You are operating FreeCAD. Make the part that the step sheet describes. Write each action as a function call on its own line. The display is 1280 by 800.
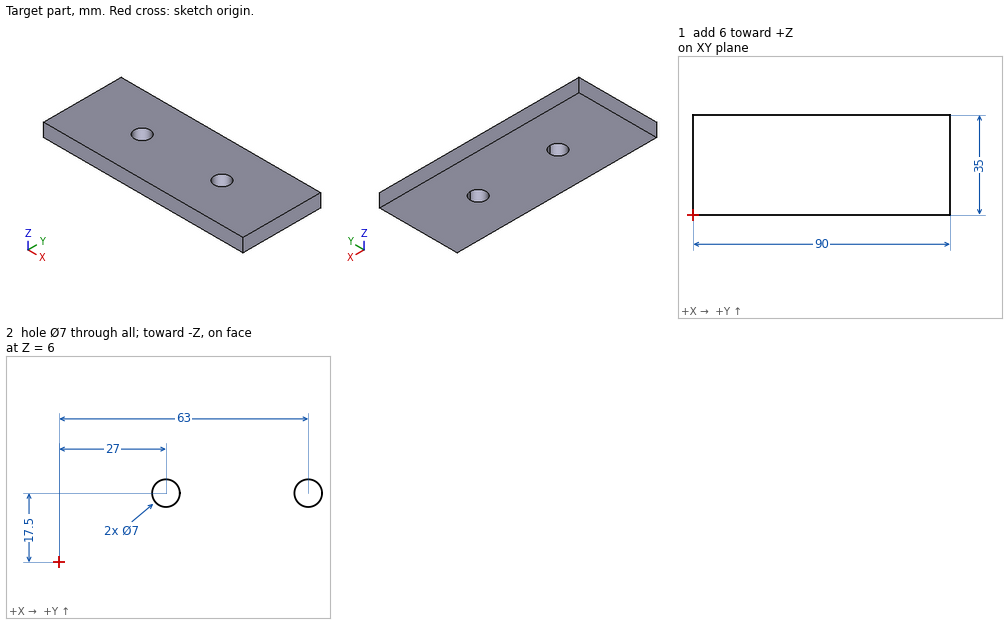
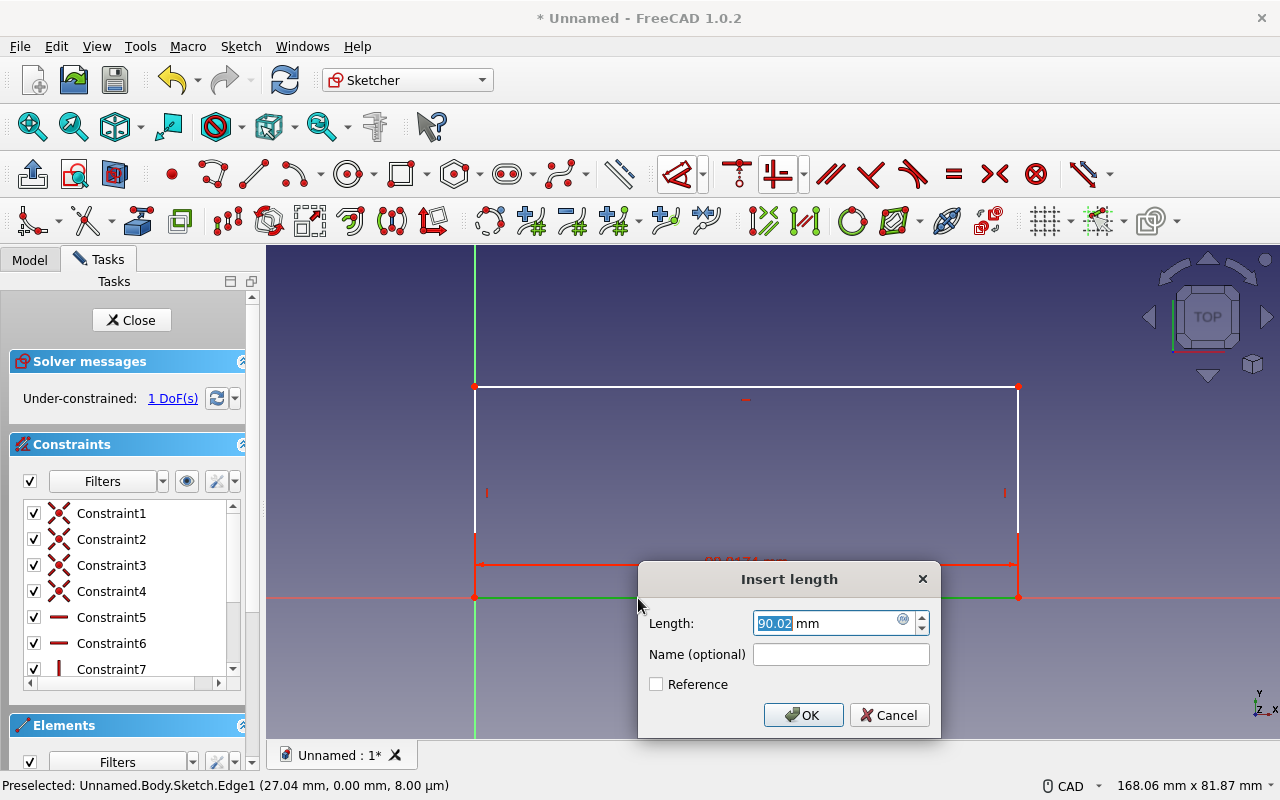
text(90)
key(Return)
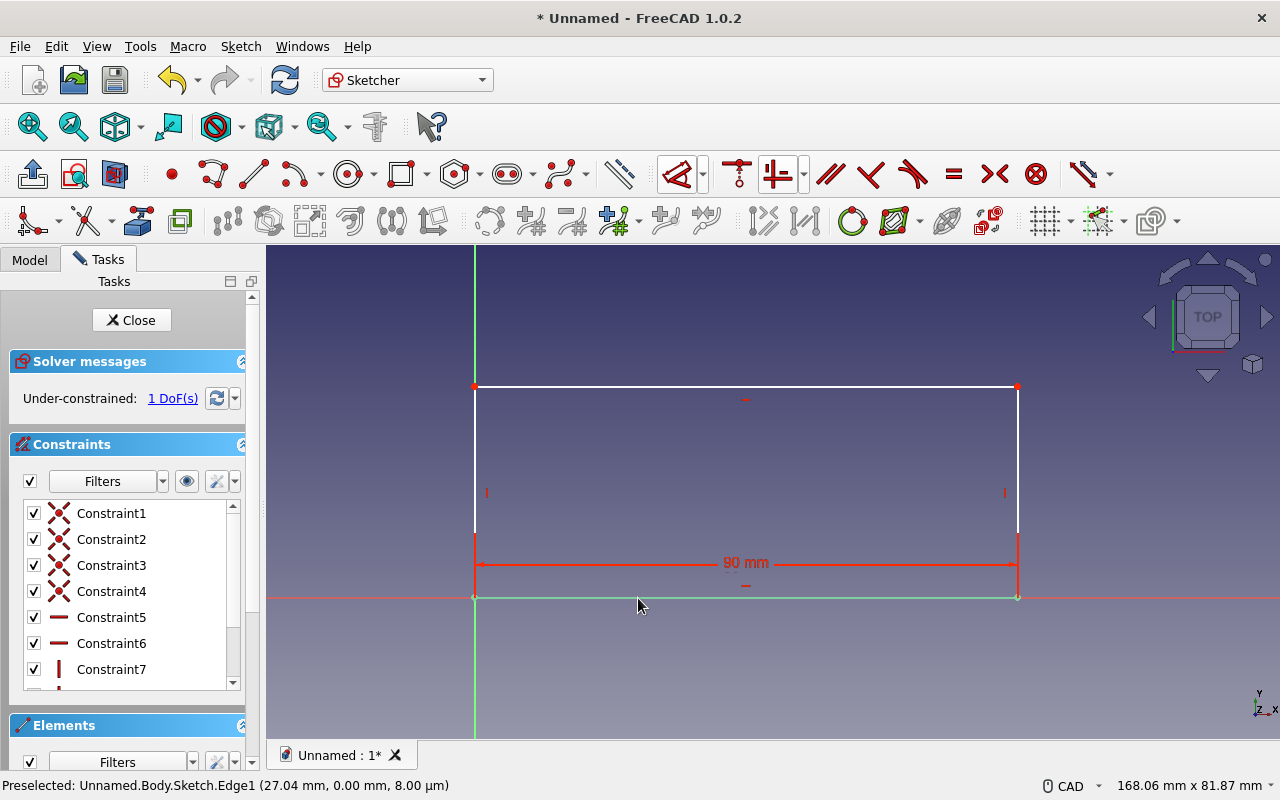
click(1018, 534)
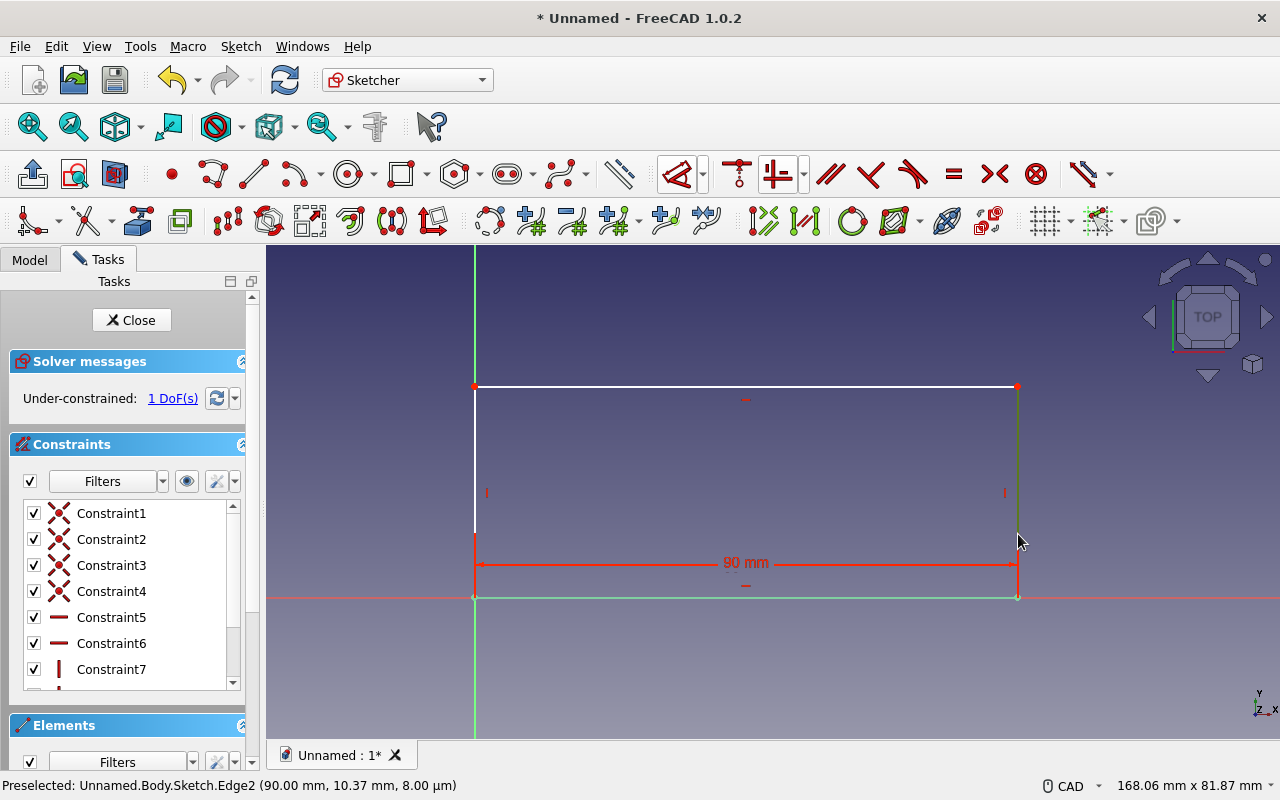
key(i)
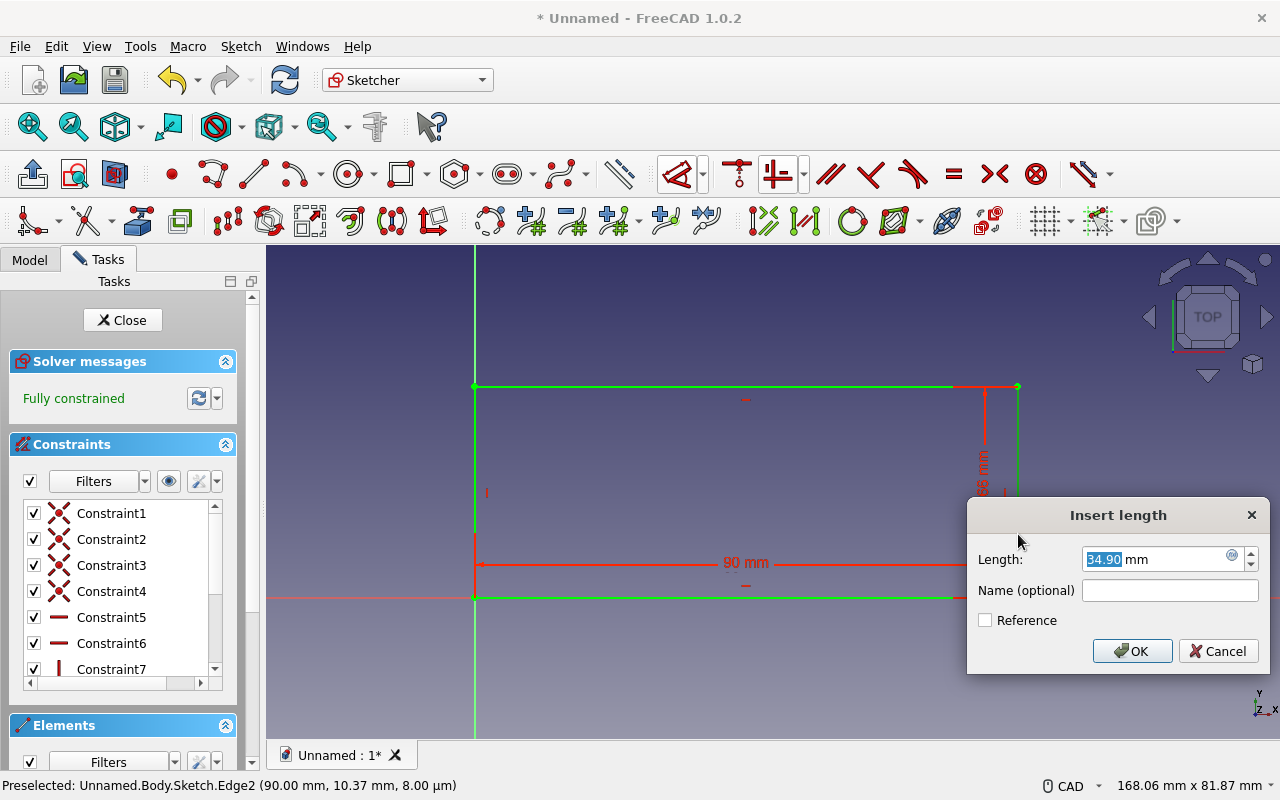
text(35)
key(Return)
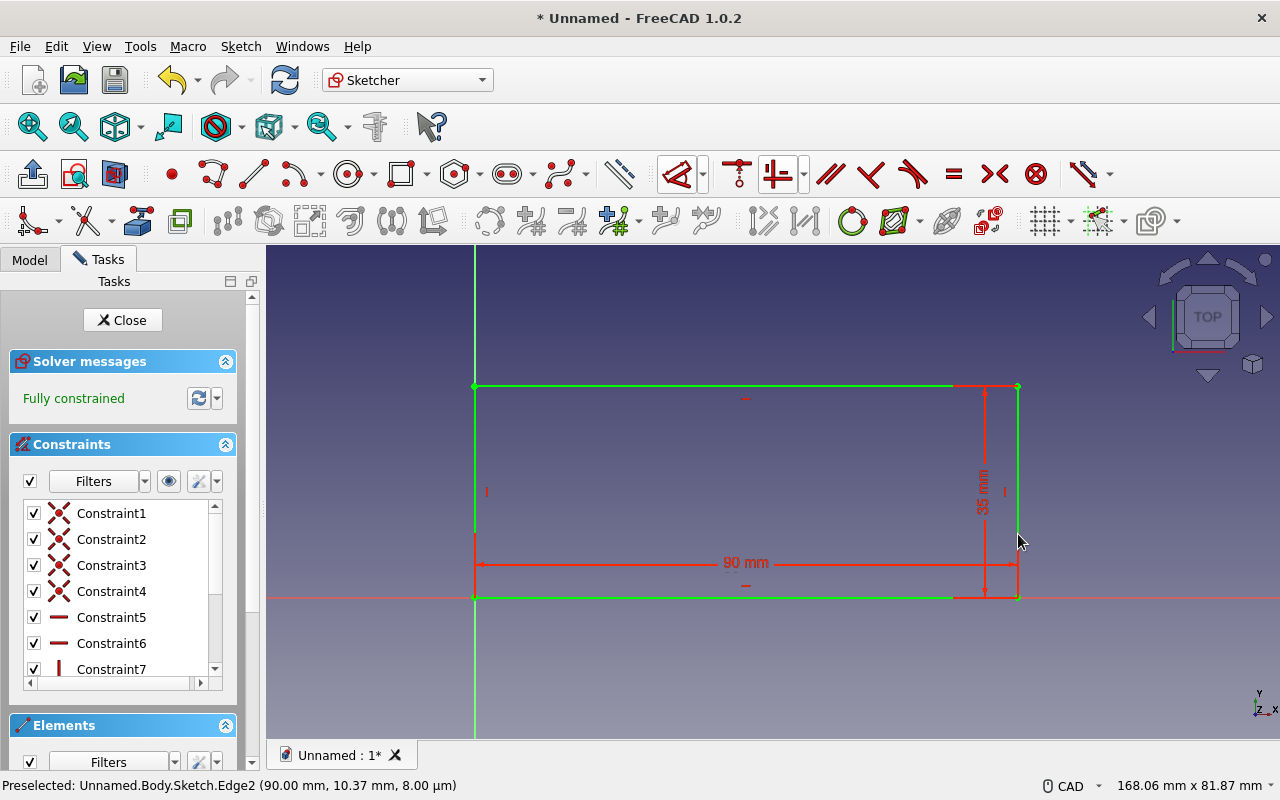
click(123, 320)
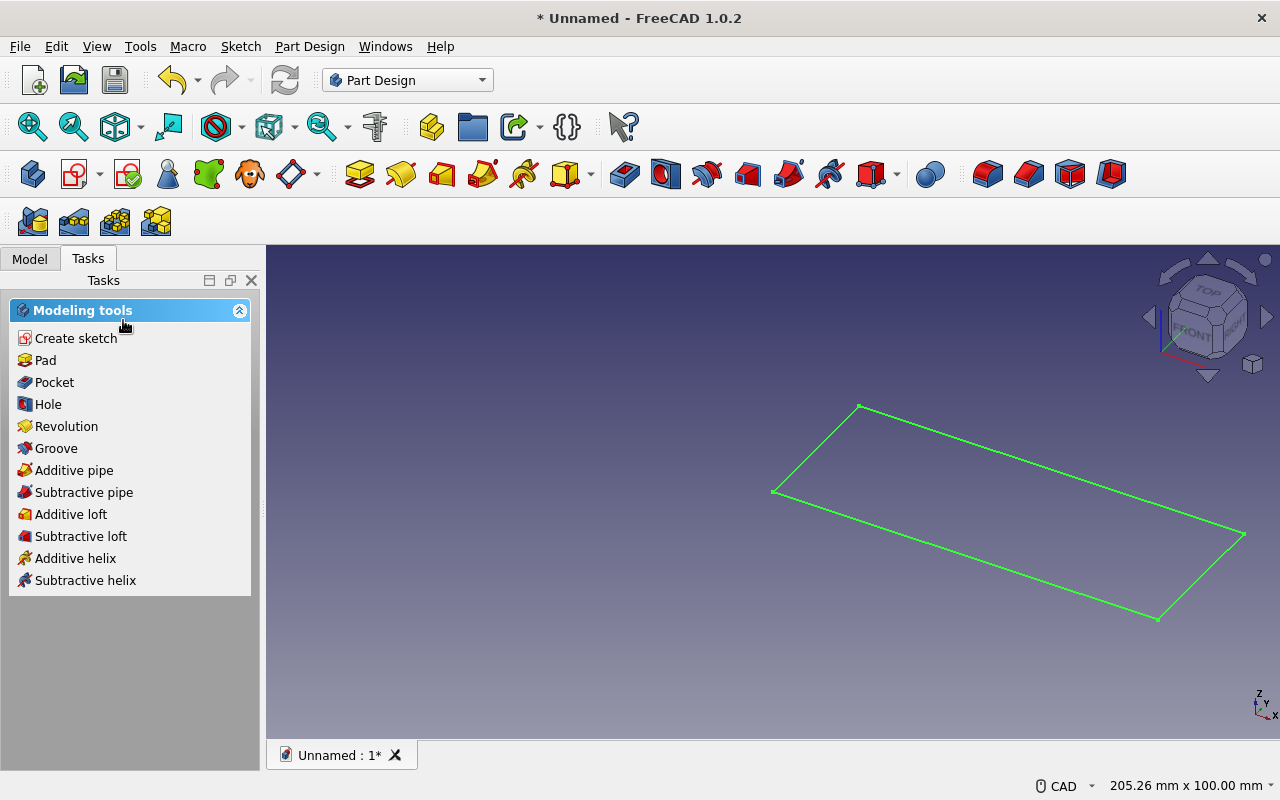
click(360, 174)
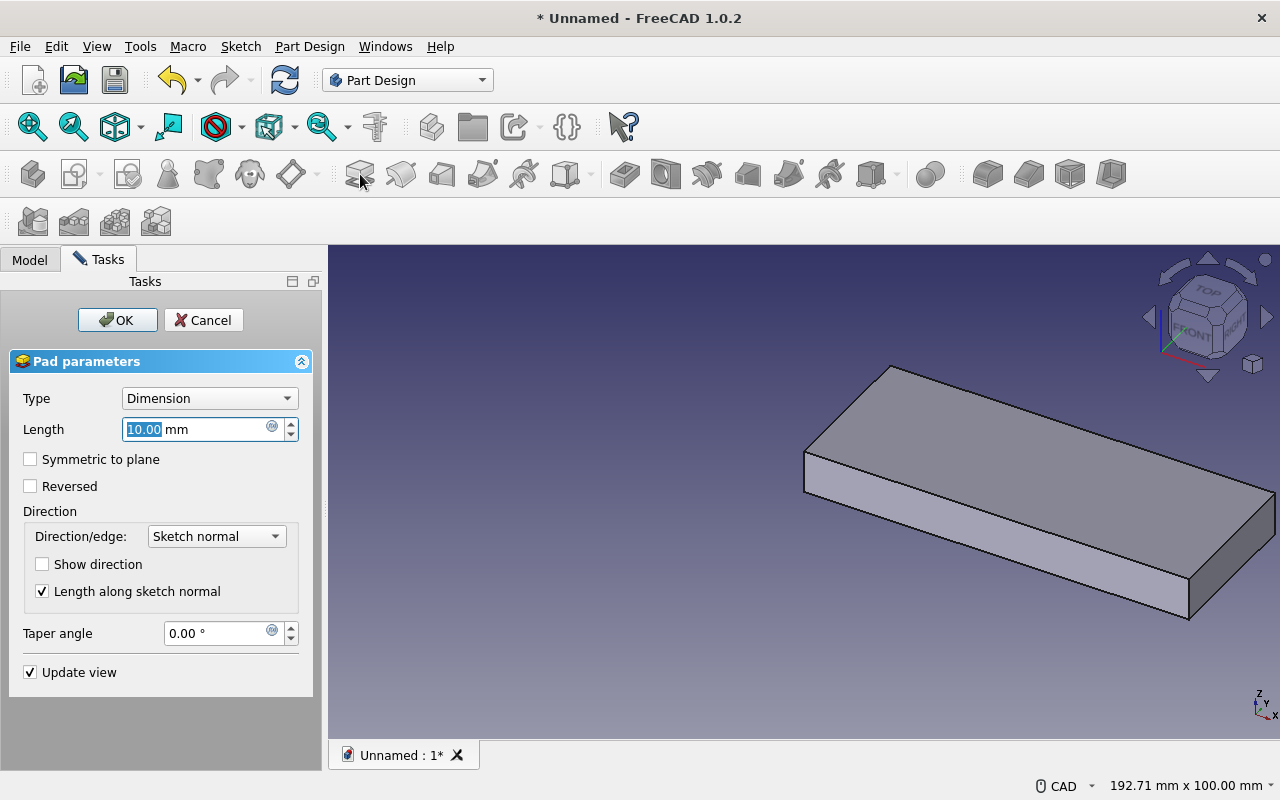
text(6)
key(Tab)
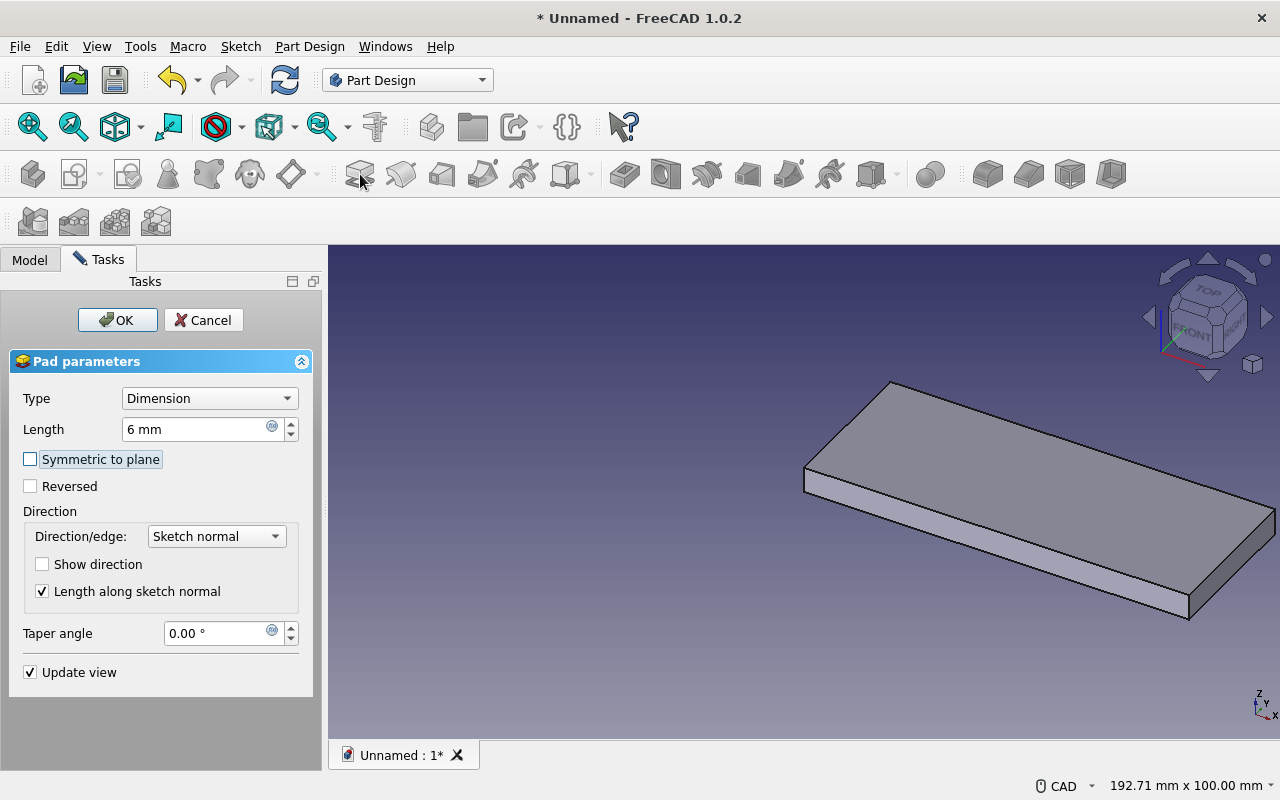
click(118, 320)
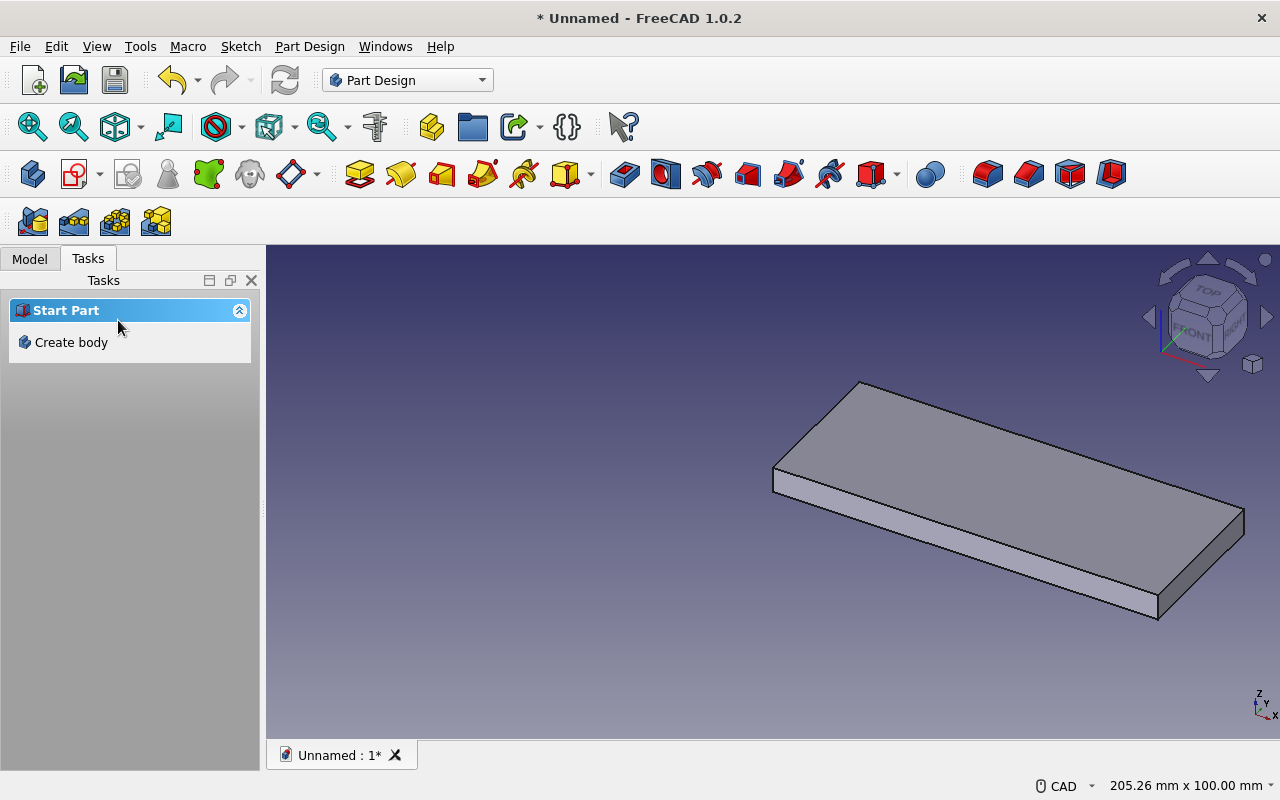
click(1119, 524)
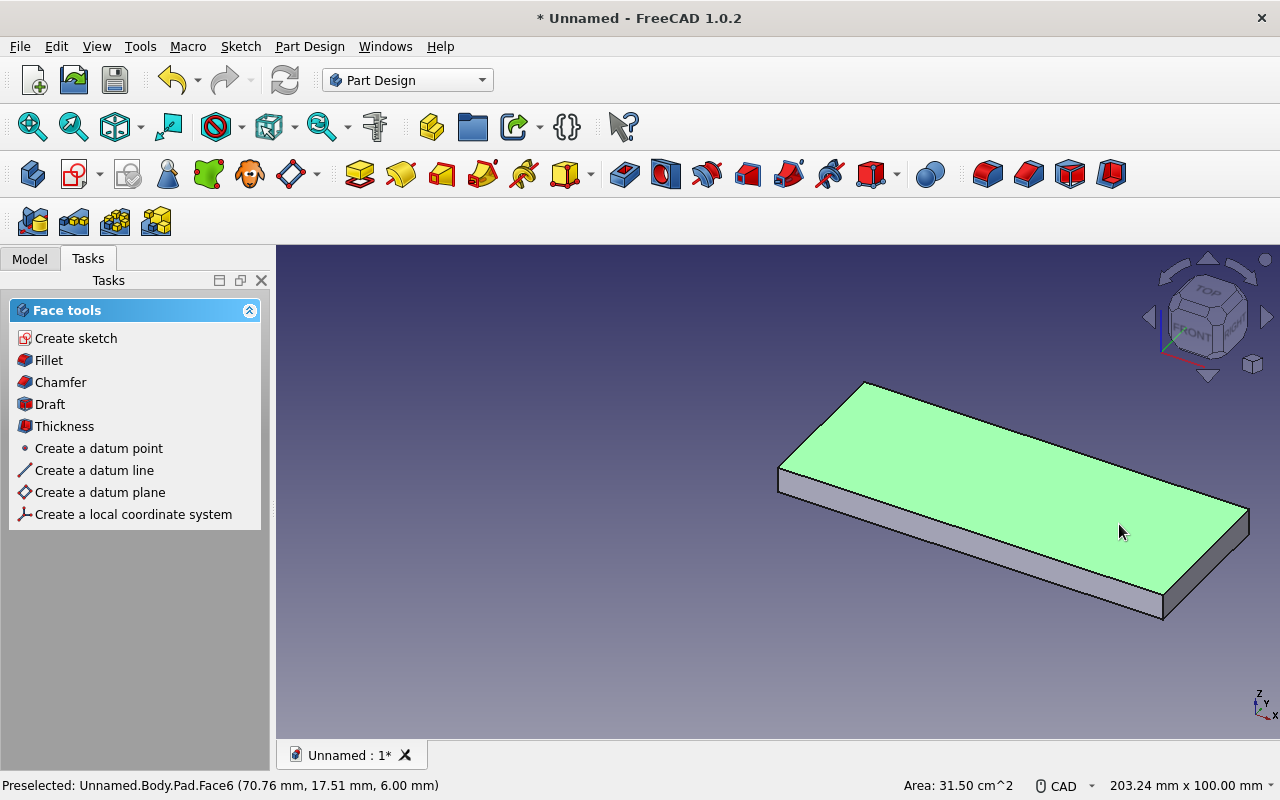
click(74, 174)